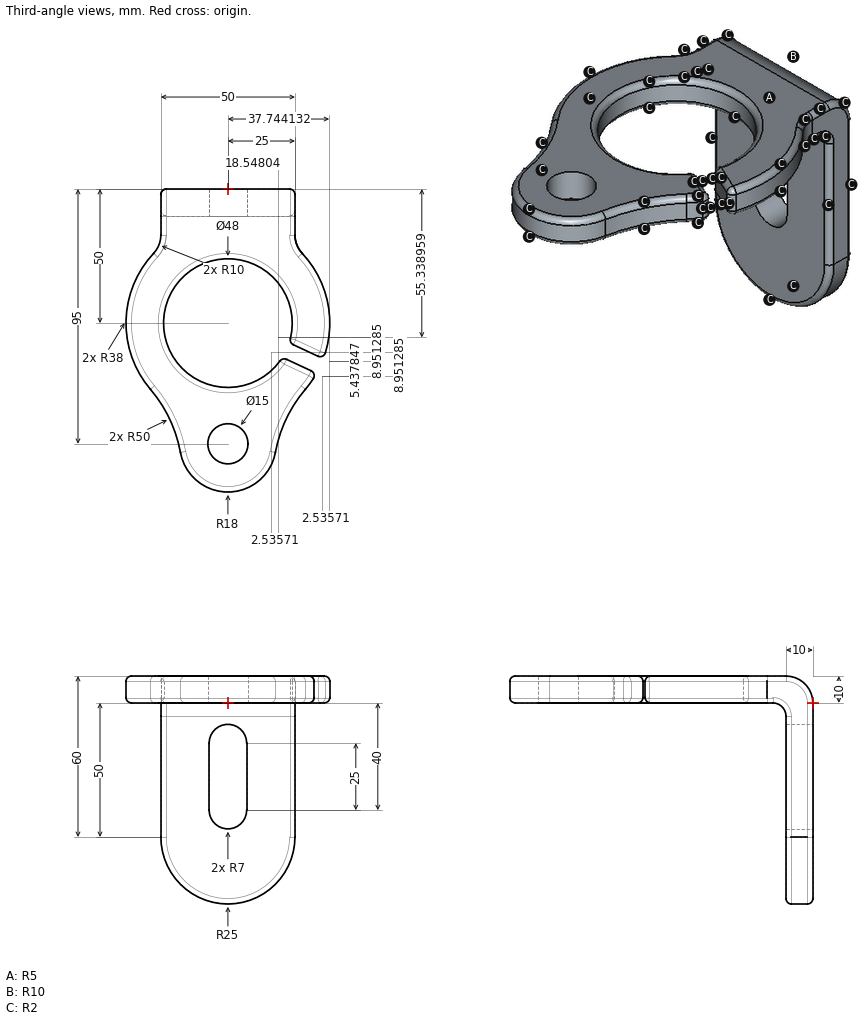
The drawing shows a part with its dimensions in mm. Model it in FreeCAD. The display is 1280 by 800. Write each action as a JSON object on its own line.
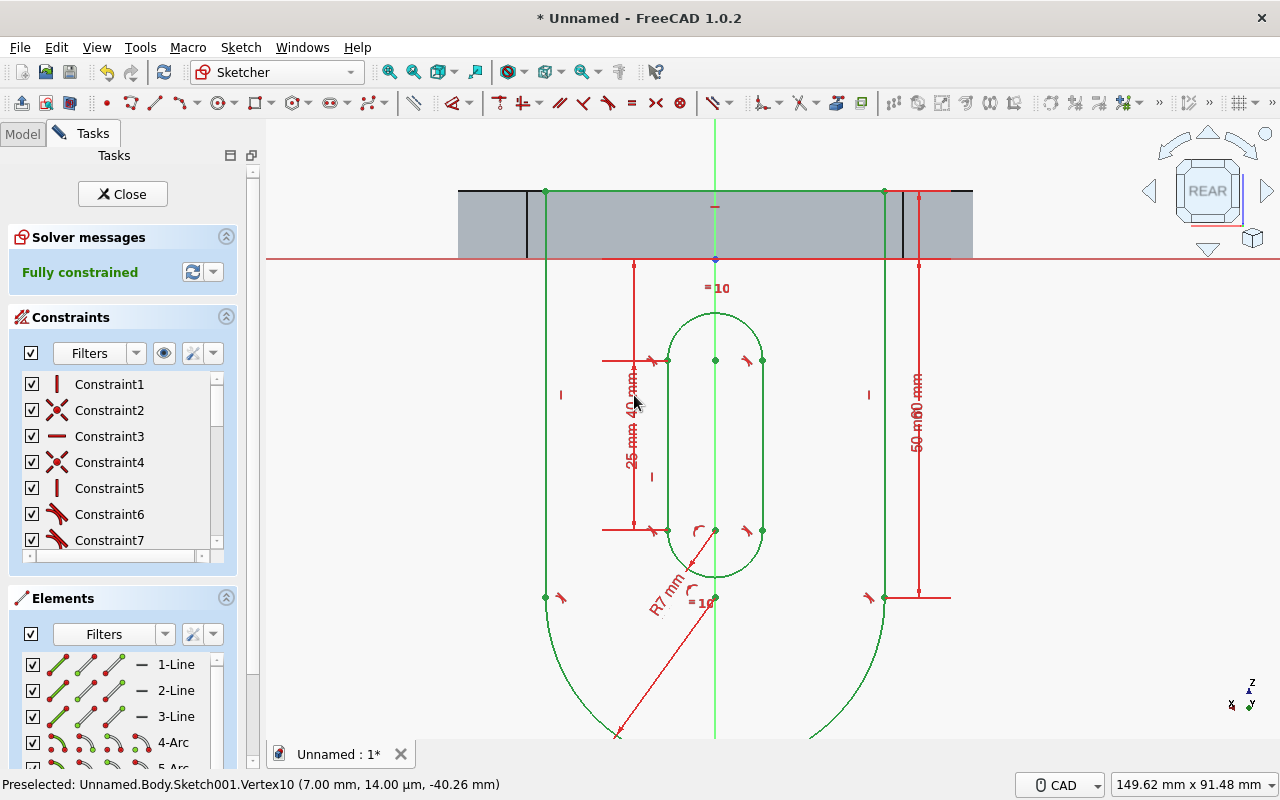
{"action": "left_click", "coordinate": [123, 194]}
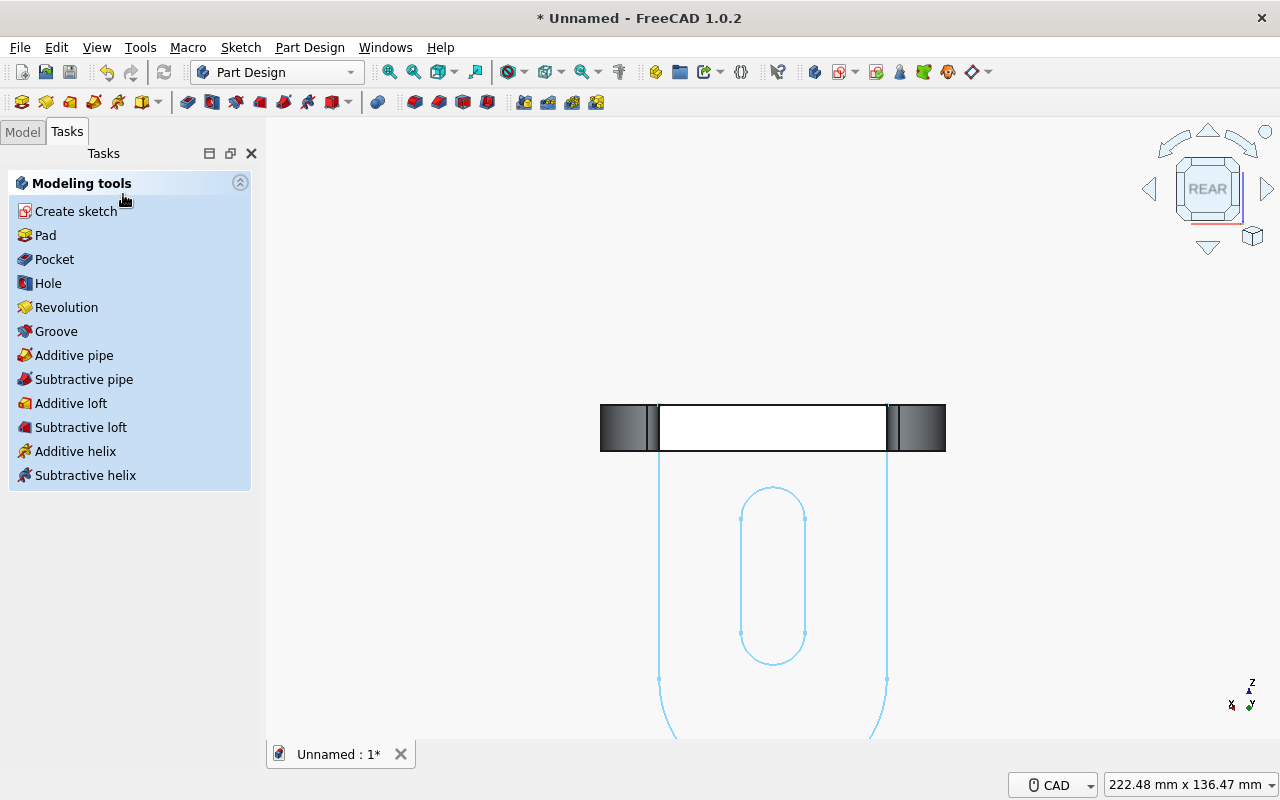
{"action": "left_click", "coordinate": [22, 102]}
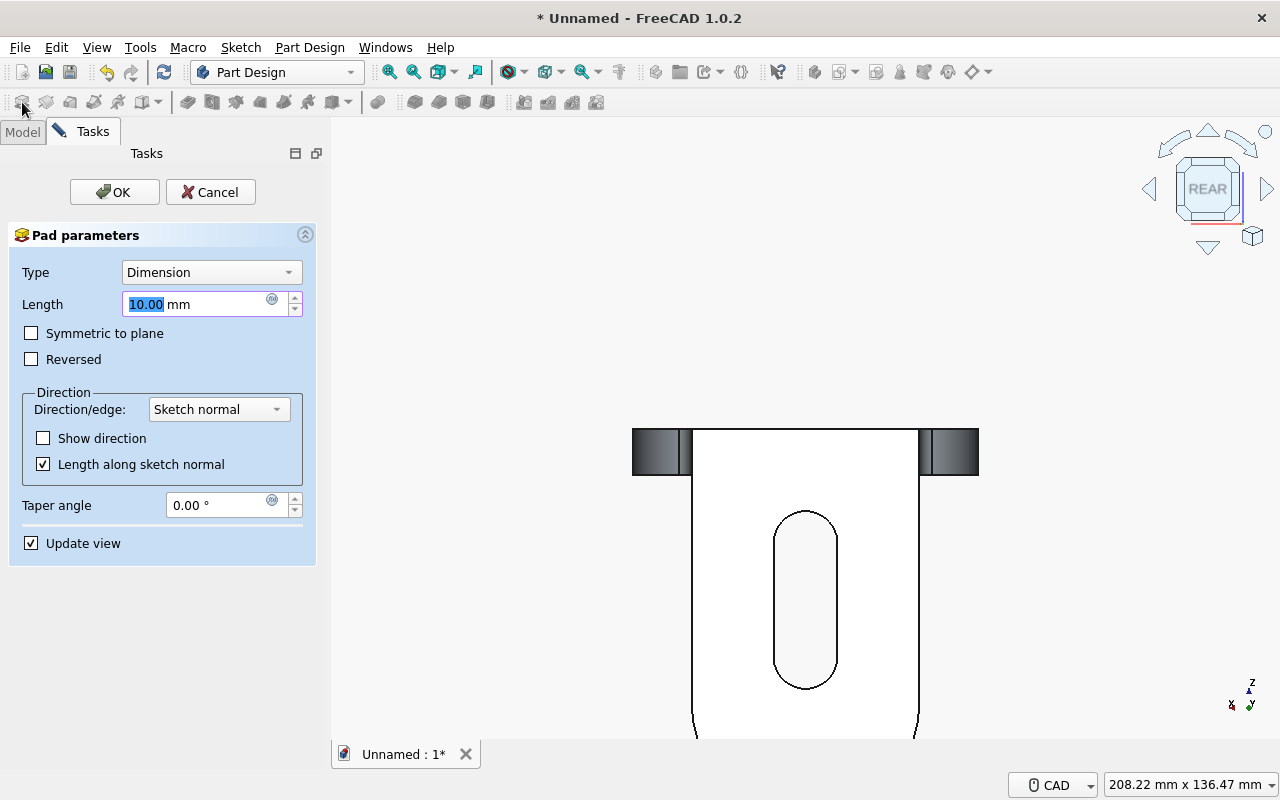
{"action": "type", "text": "10"}
{"action": "key", "text": "Tab"}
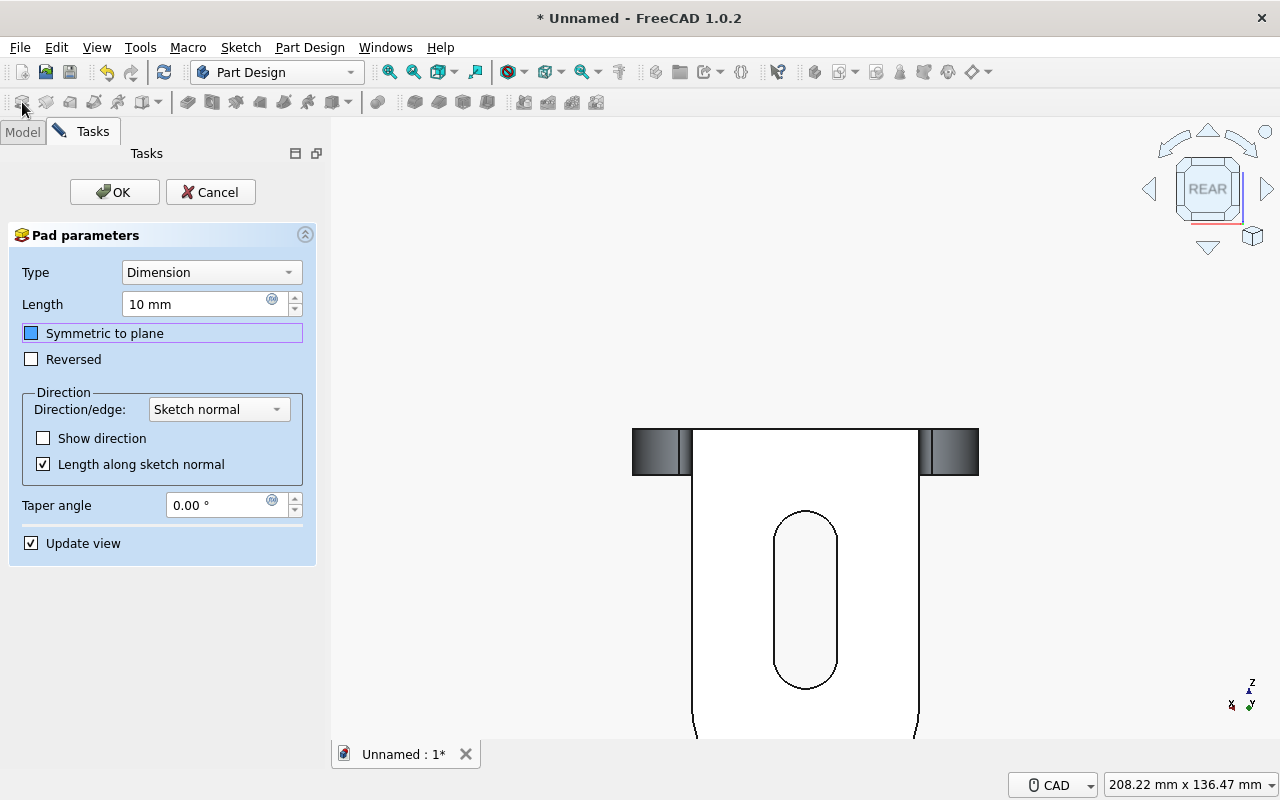
{"action": "left_click", "coordinate": [30, 359]}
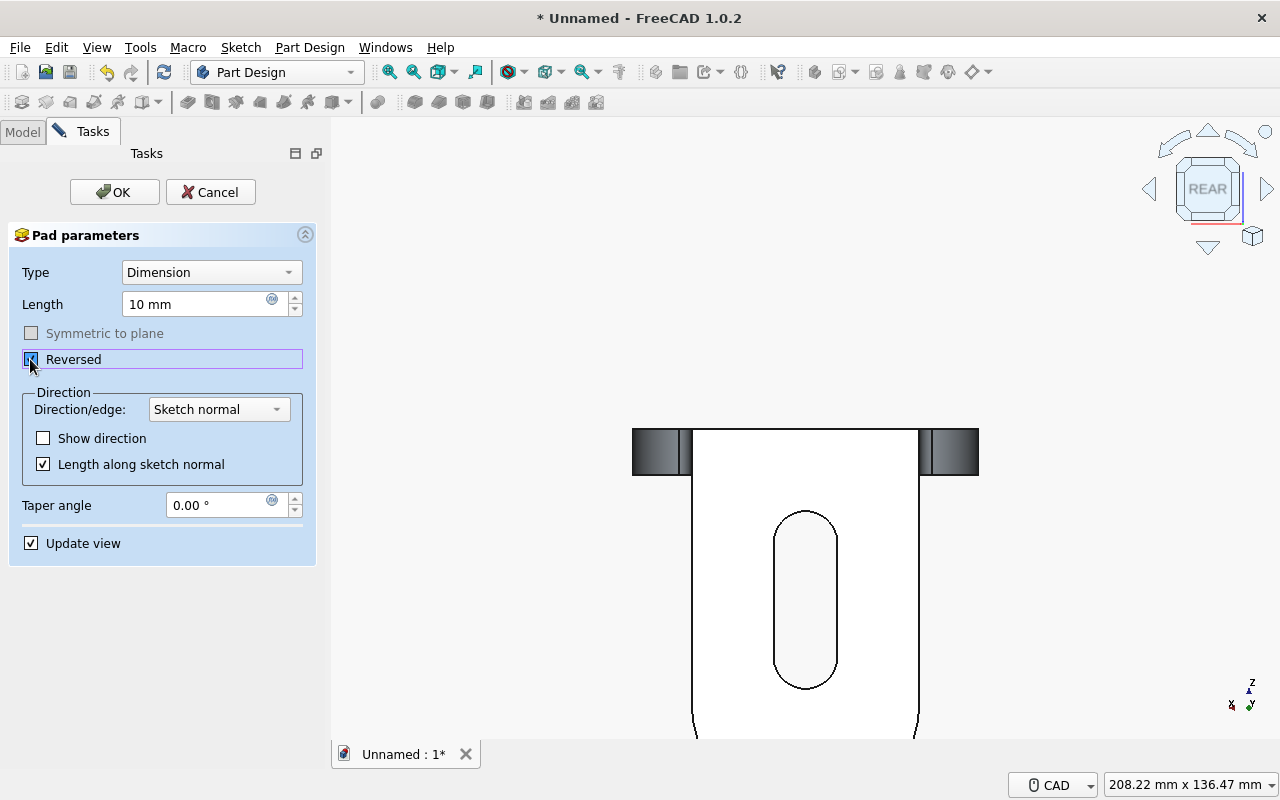
{"action": "left_click", "coordinate": [115, 192]}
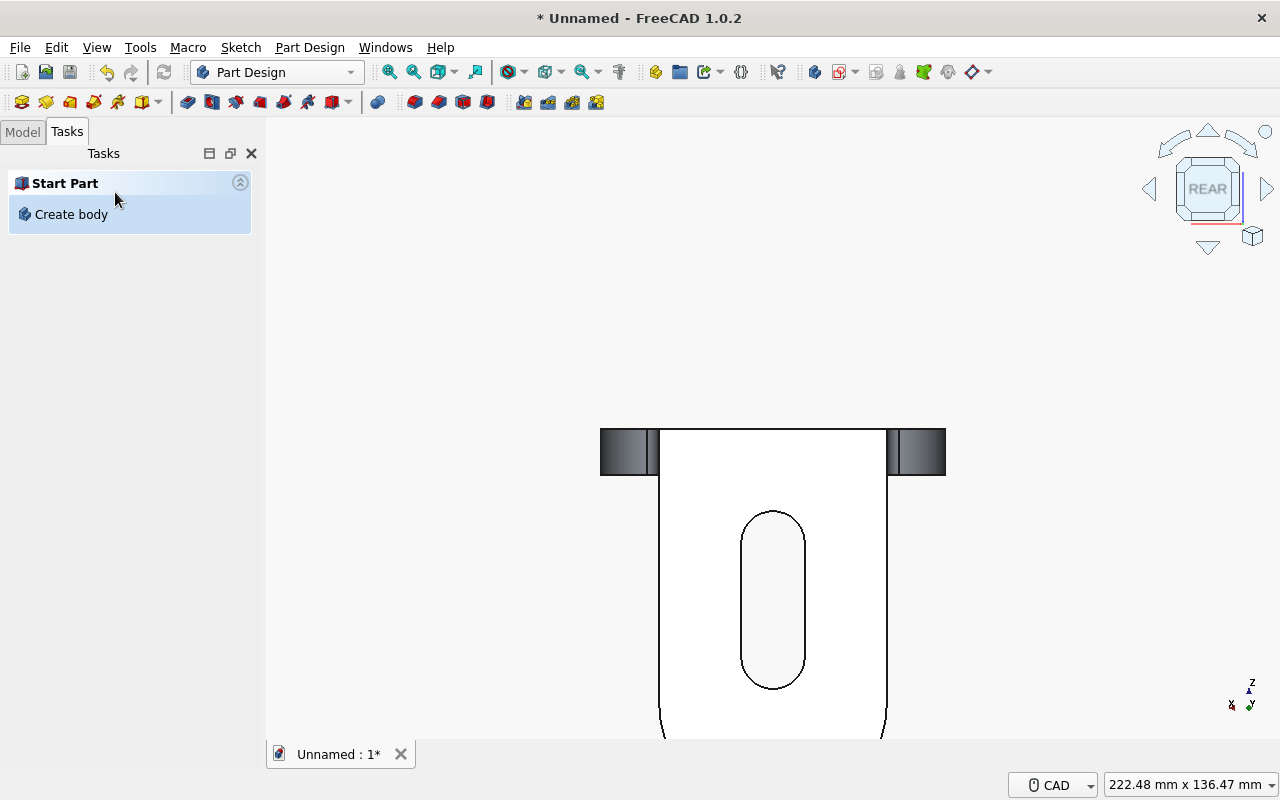
{"action": "left_click", "coordinate": [390, 72]}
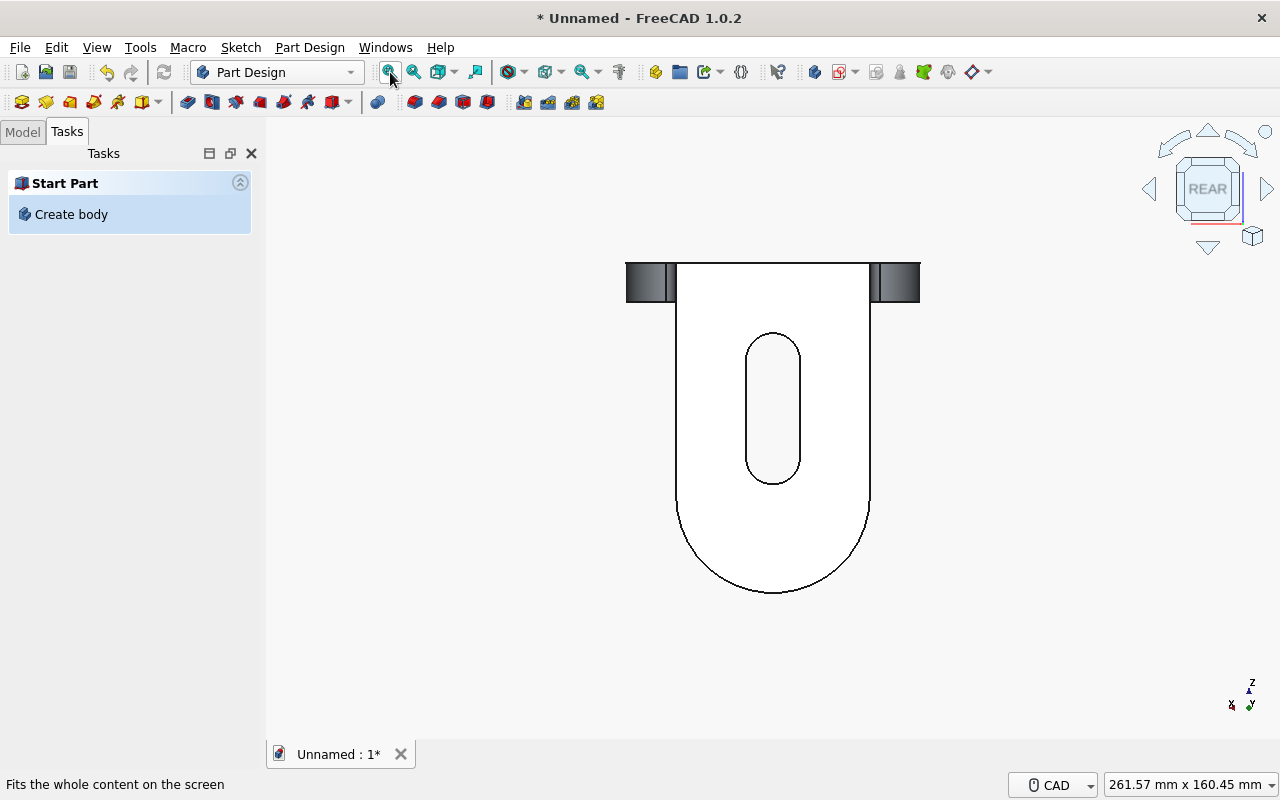
{"action": "left_click", "coordinate": [840, 72]}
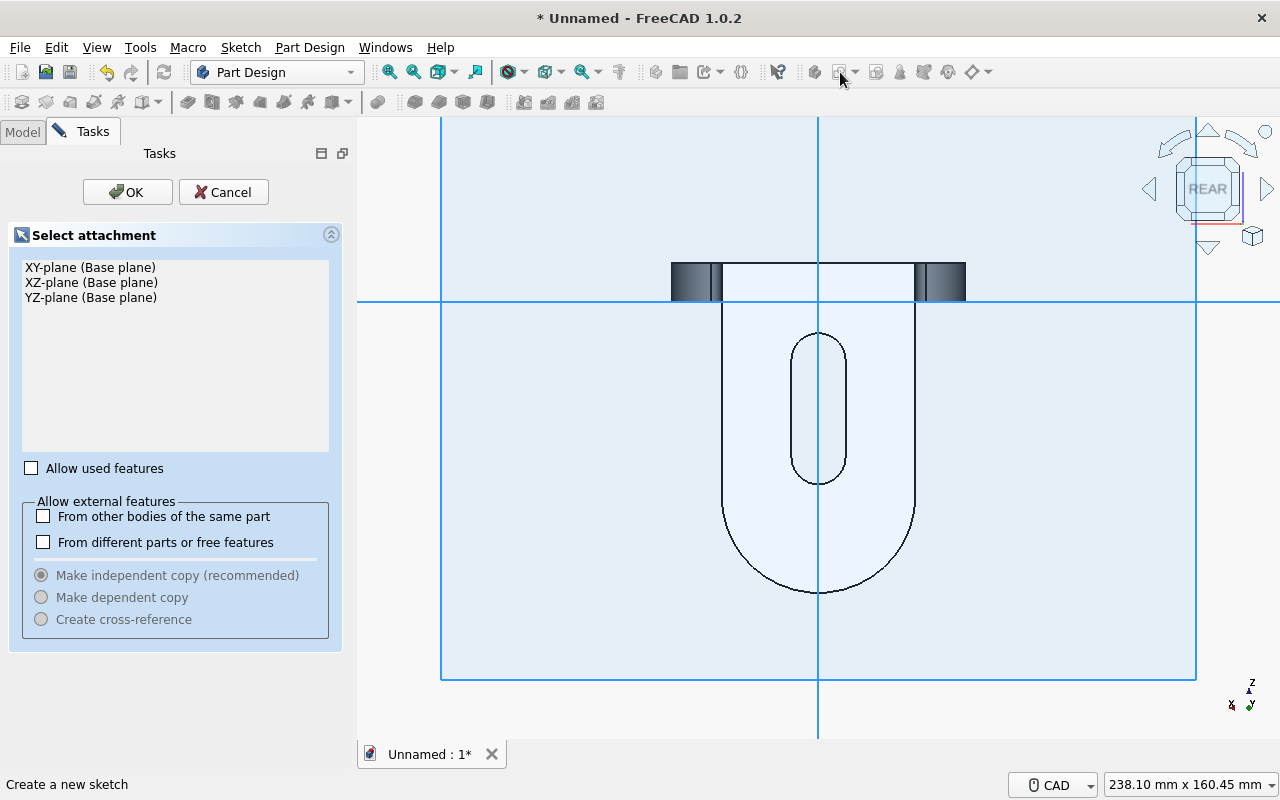
{"action": "left_click", "coordinate": [82, 268]}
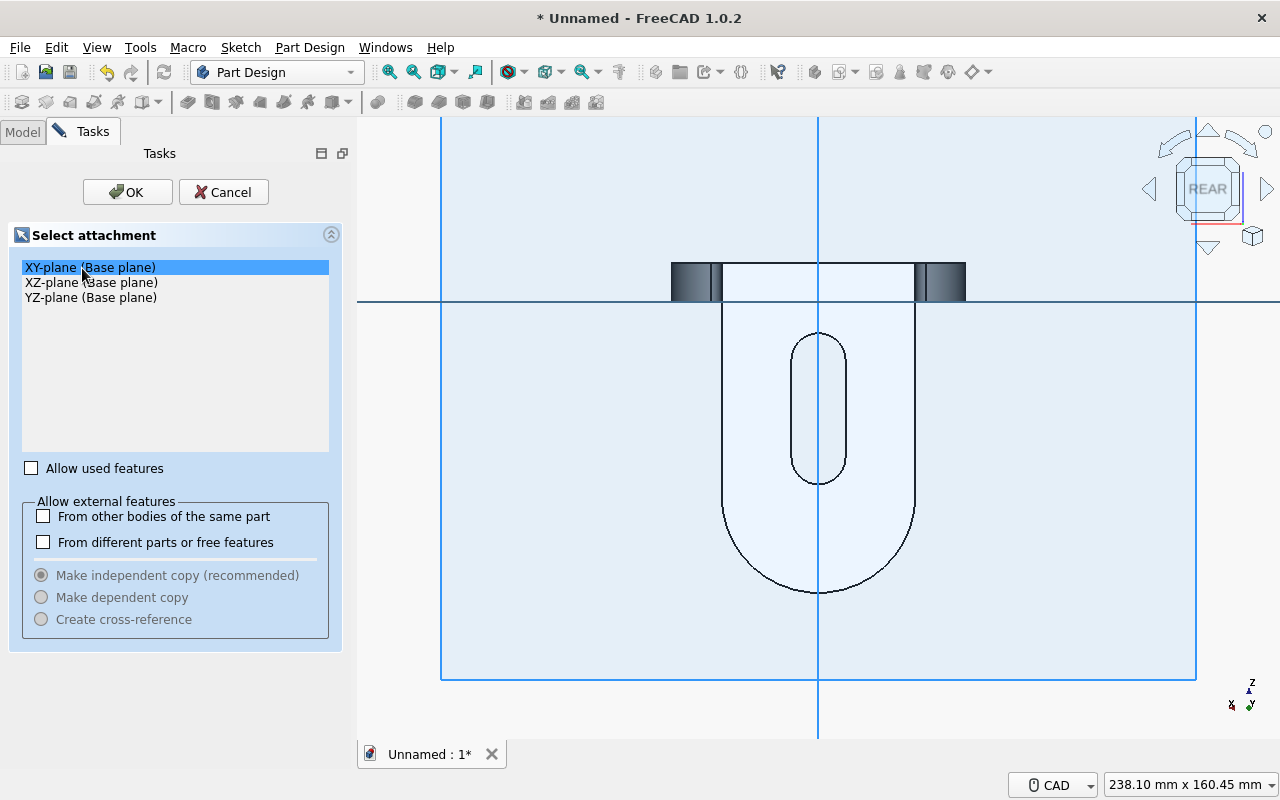
{"action": "left_click", "coordinate": [128, 192]}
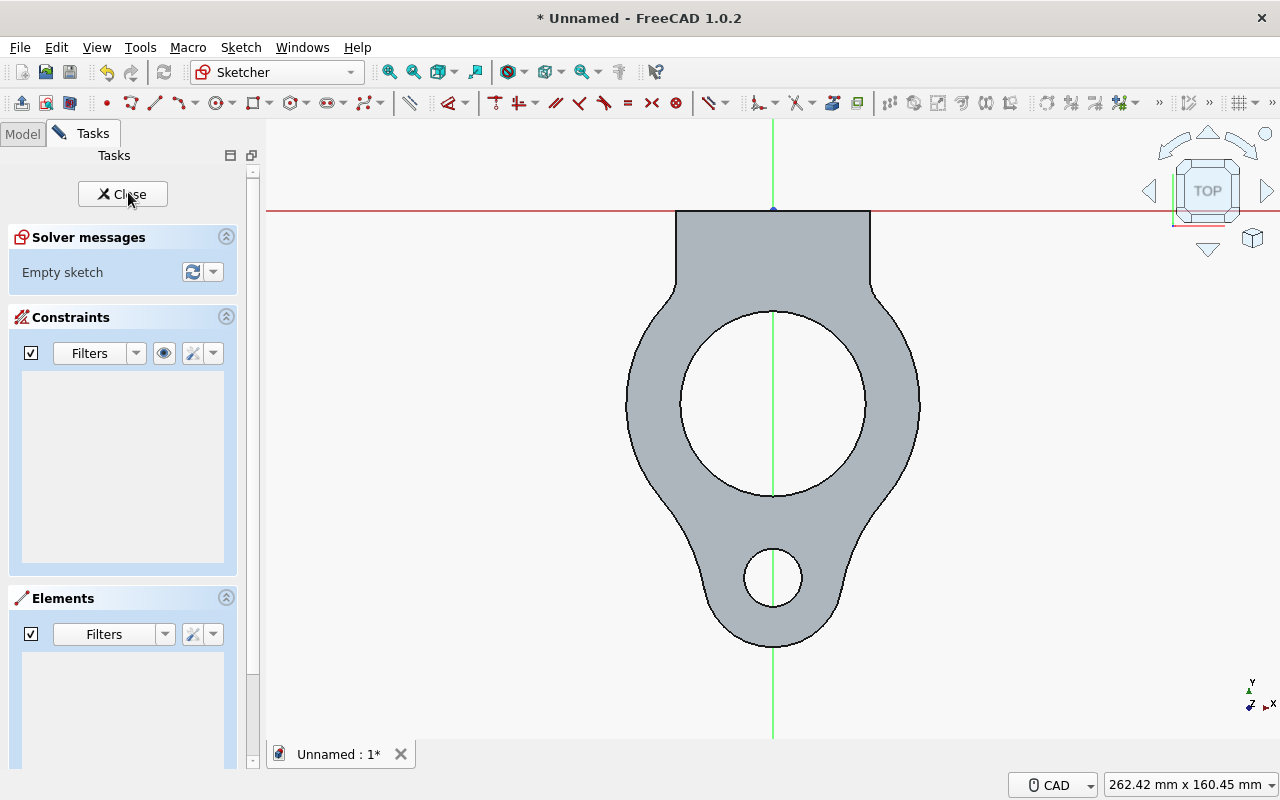
{"action": "left_click", "coordinate": [70, 104]}